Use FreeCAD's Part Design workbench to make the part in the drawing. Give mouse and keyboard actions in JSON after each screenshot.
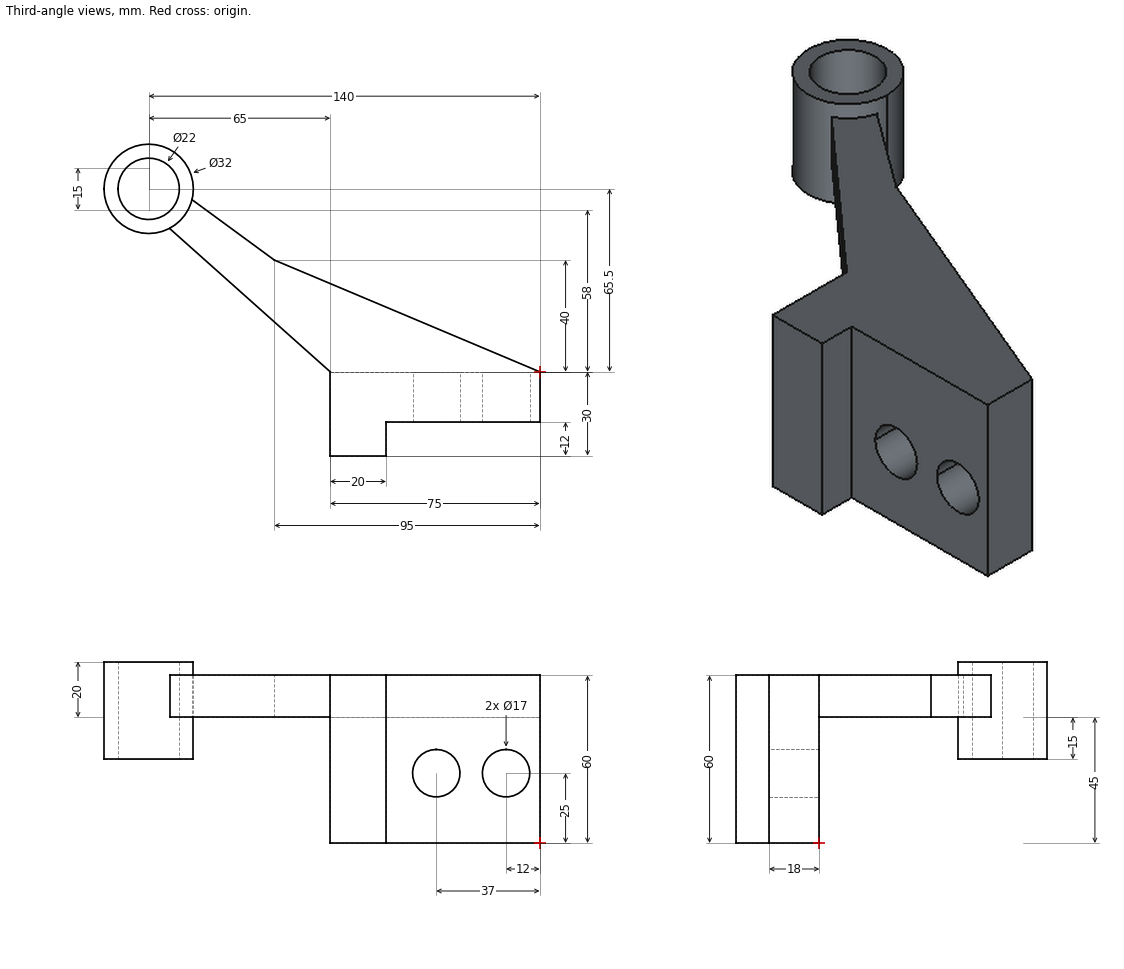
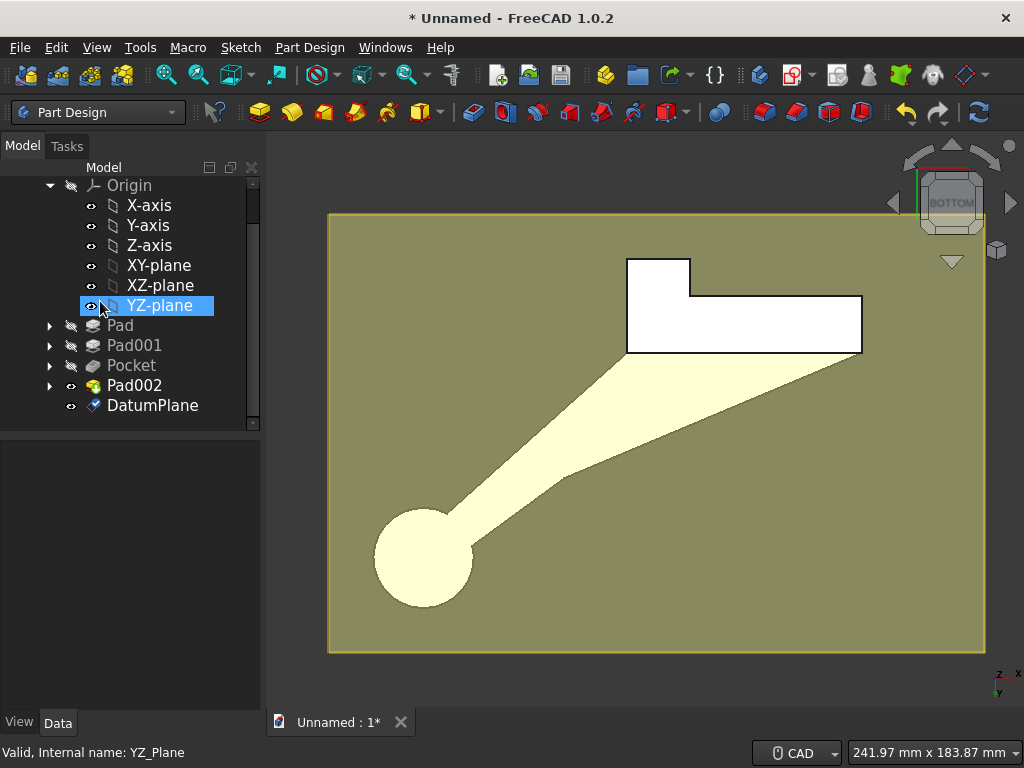
{"action": "left_click", "coordinate": [116, 406]}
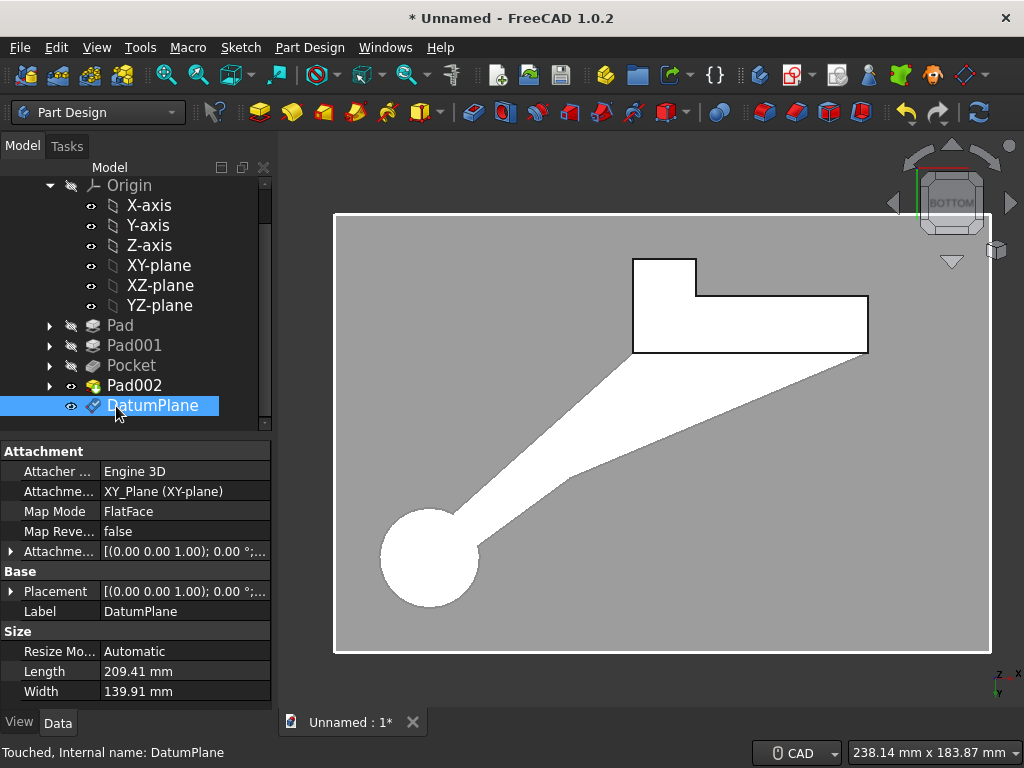
{"action": "left_click", "coordinate": [792, 76]}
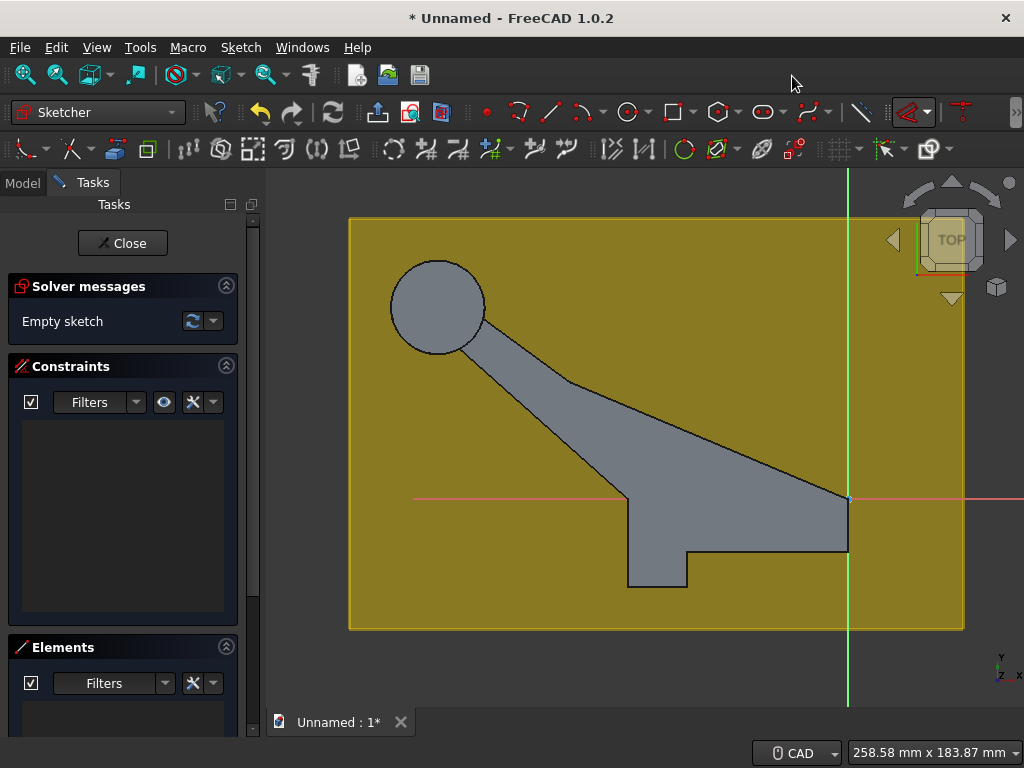
{"action": "left_click", "coordinate": [442, 112]}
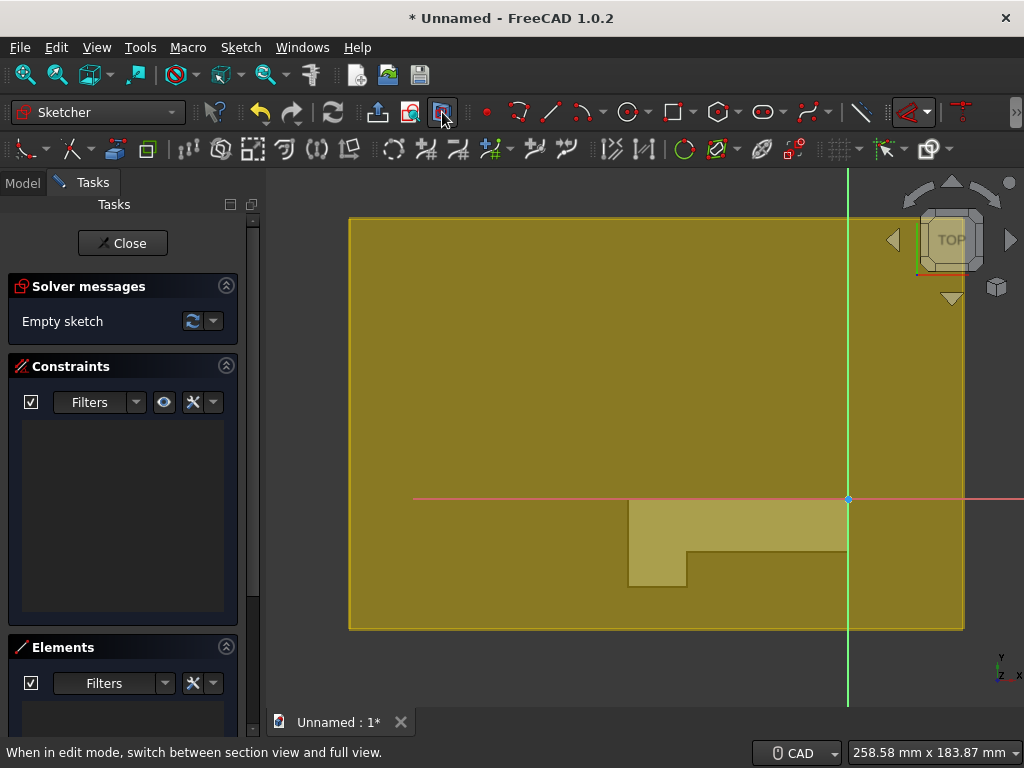
{"action": "scroll", "coordinate": [378, 251], "scroll_direction": "up", "scroll_amount": 6}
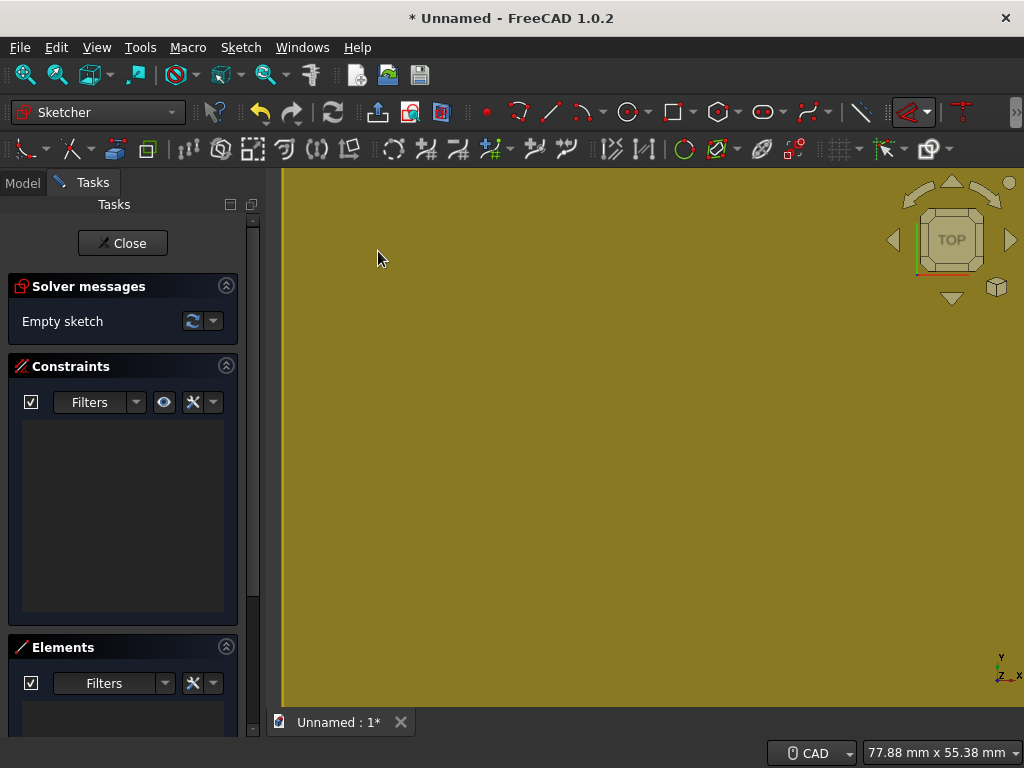
{"action": "left_click", "coordinate": [628, 112]}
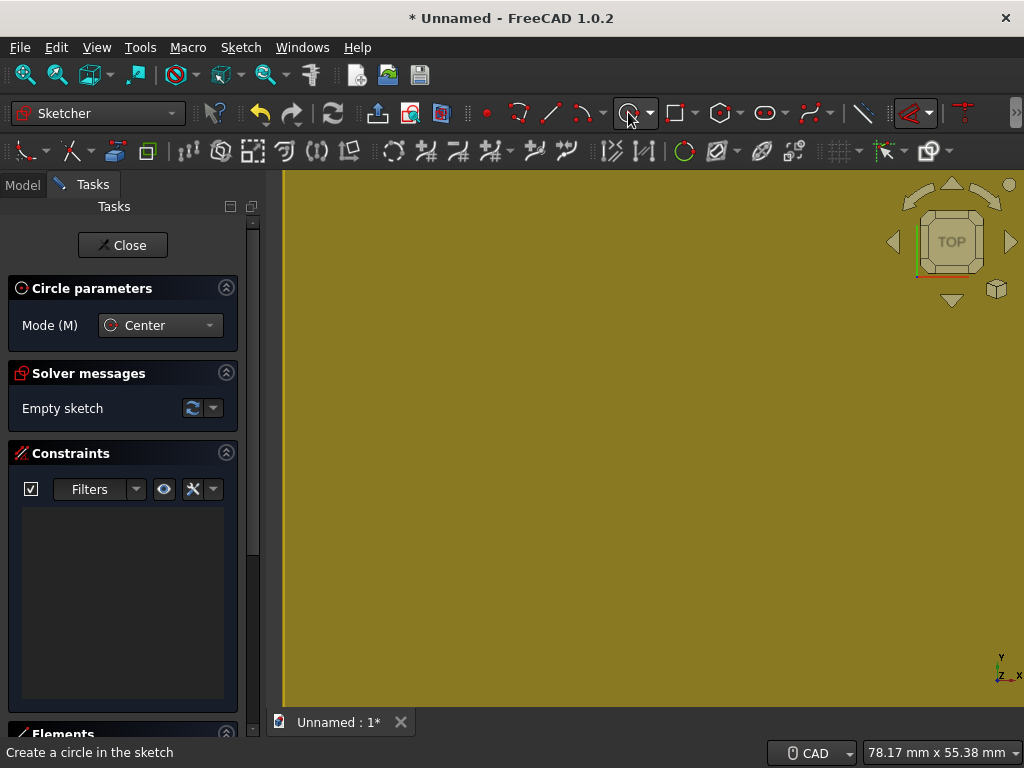
{"action": "left_click", "coordinate": [576, 439]}
{"action": "left_click", "coordinate": [686, 329]}
{"action": "key", "text": "Escape"}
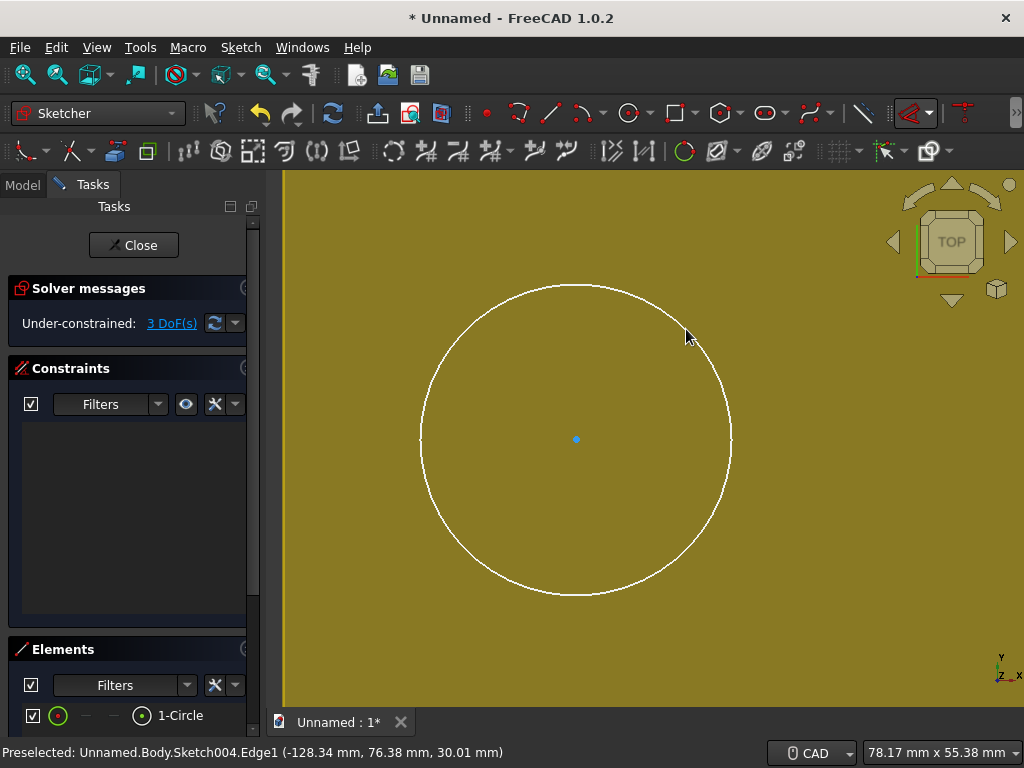
{"action": "left_click", "coordinate": [686, 330]}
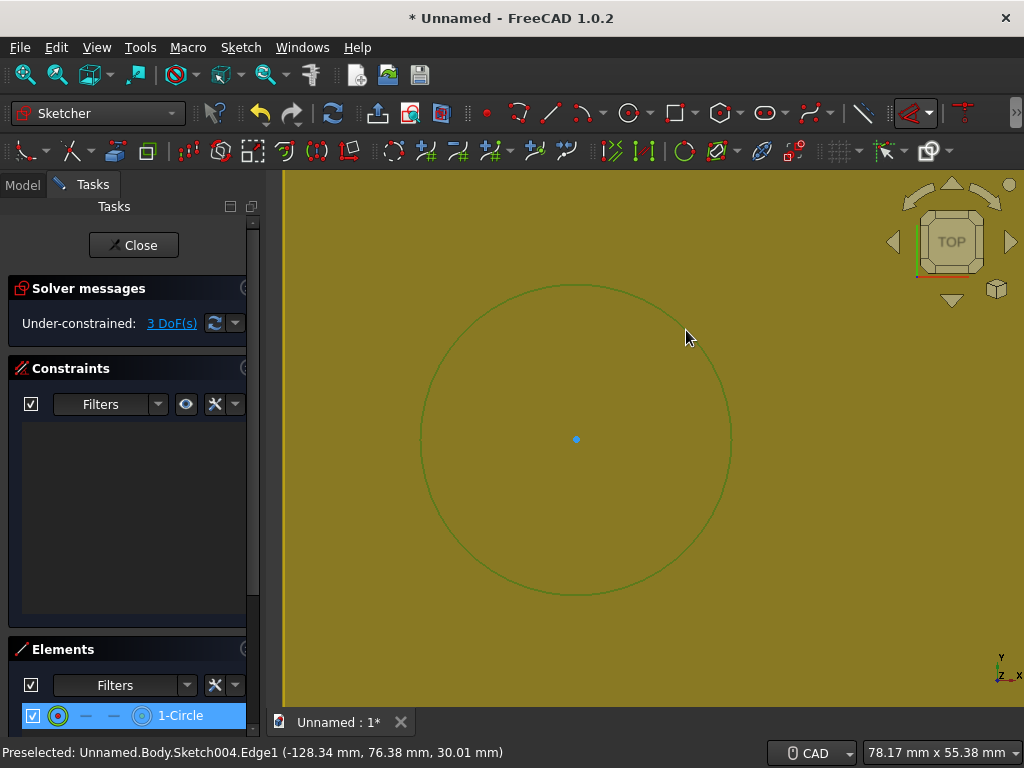
{"action": "left_click", "coordinate": [932, 114]}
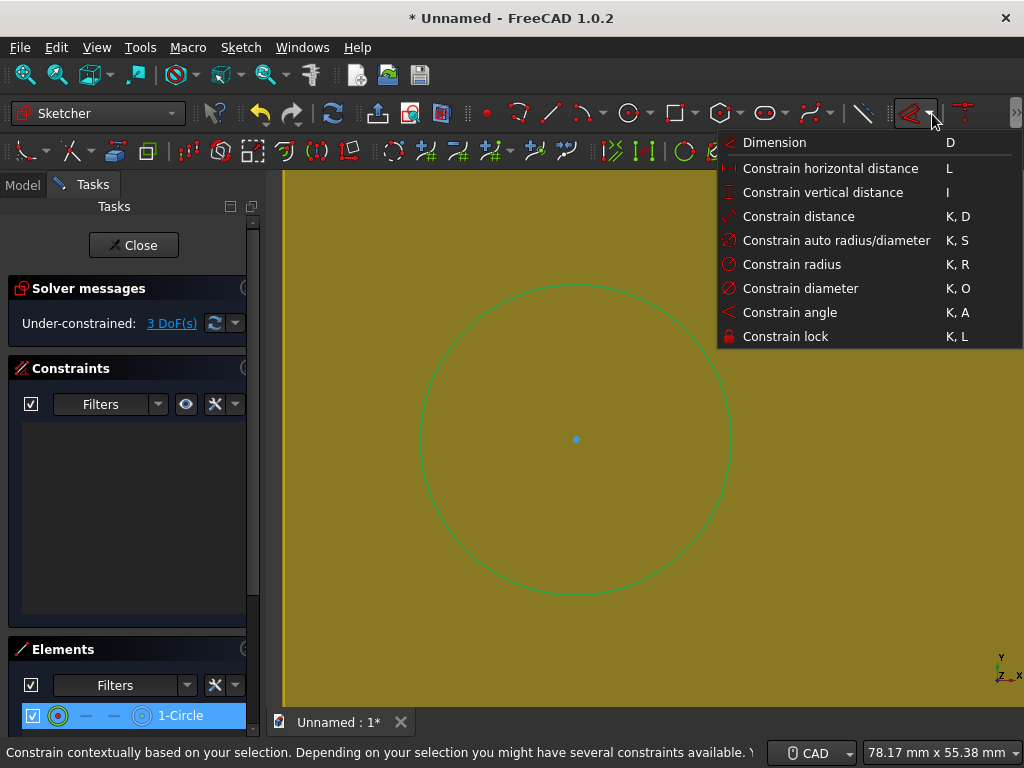
{"action": "left_click", "coordinate": [870, 288]}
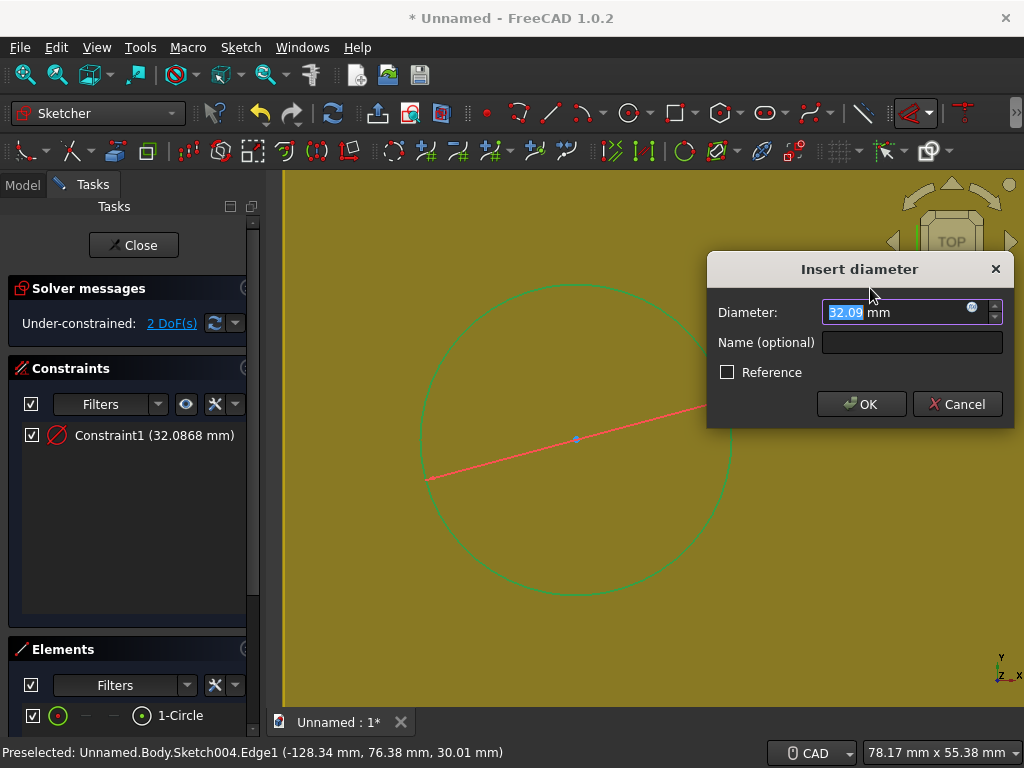
{"action": "type", "text": "32"}
{"action": "key", "text": "Return"}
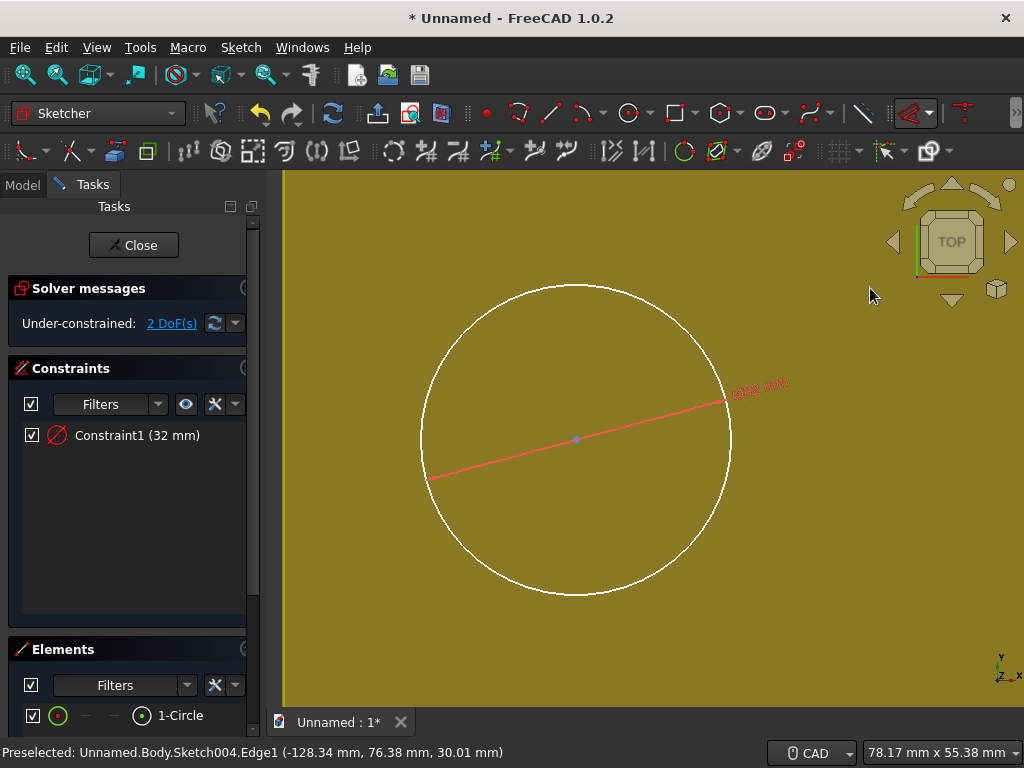
{"action": "left_click", "coordinate": [576, 440]}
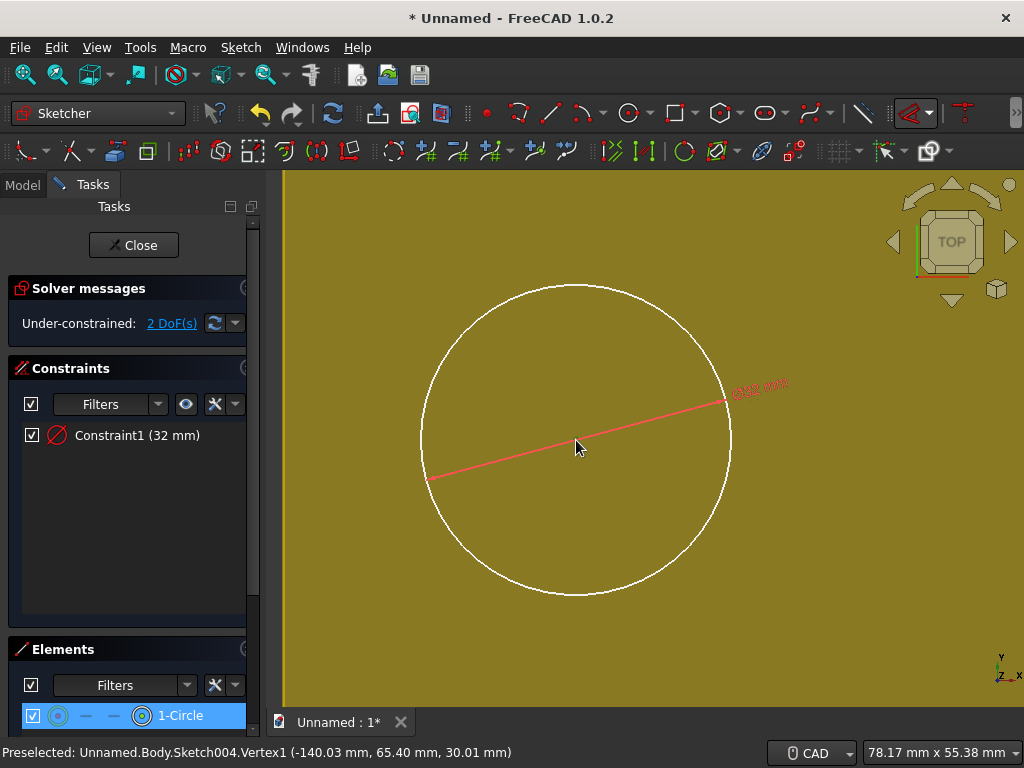
{"action": "key", "text": "l"}